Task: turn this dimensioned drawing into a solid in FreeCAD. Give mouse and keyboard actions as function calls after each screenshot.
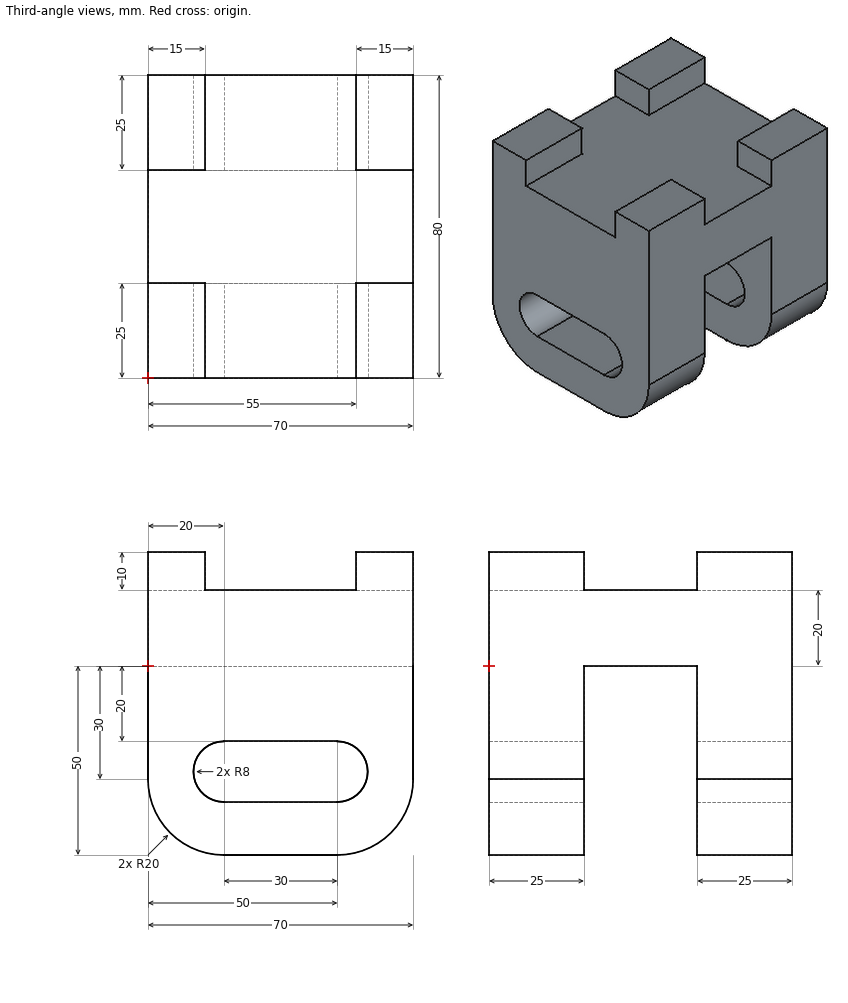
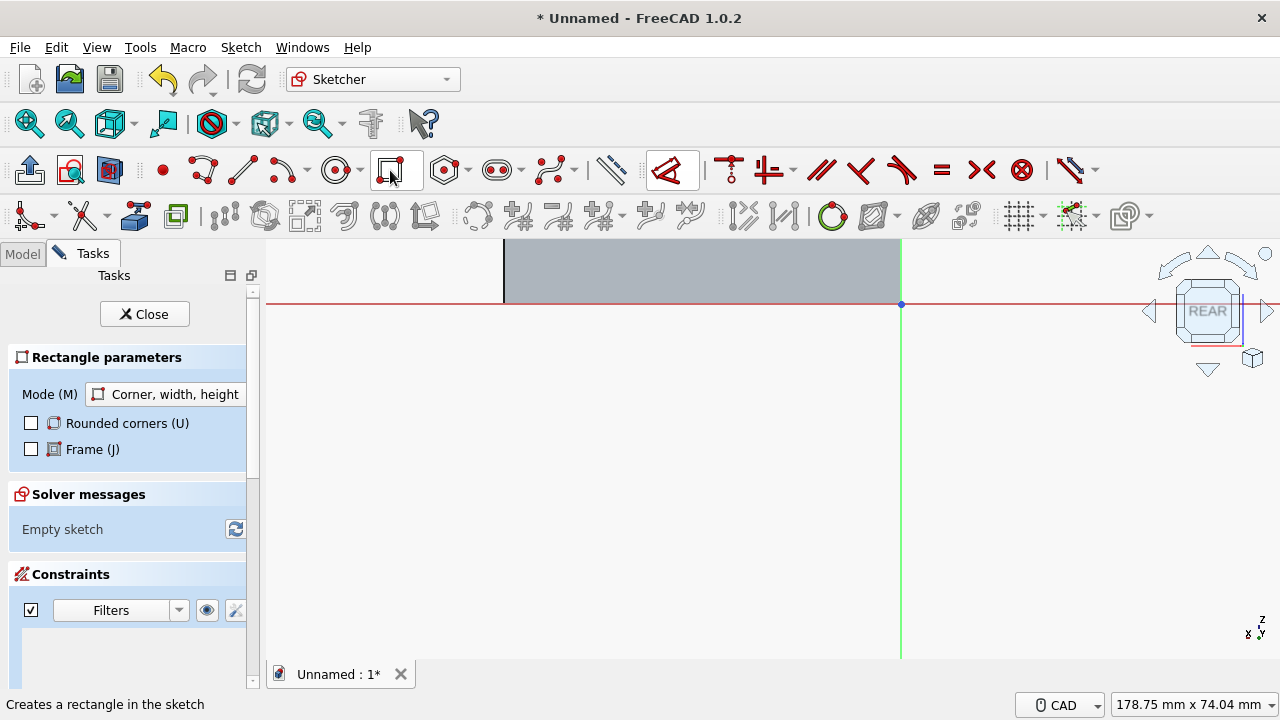
click(901, 304)
move(504, 588)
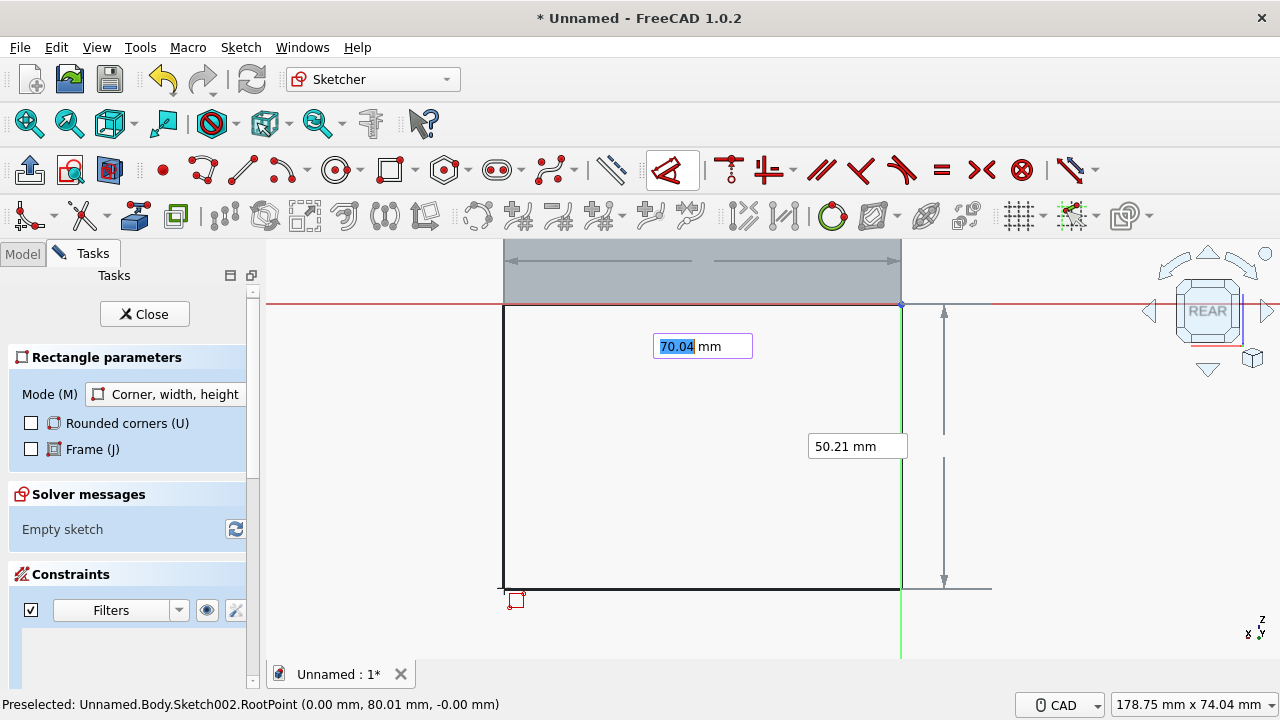
text(70)
key(Tab)
text(50)
key(Return)
key(Escape)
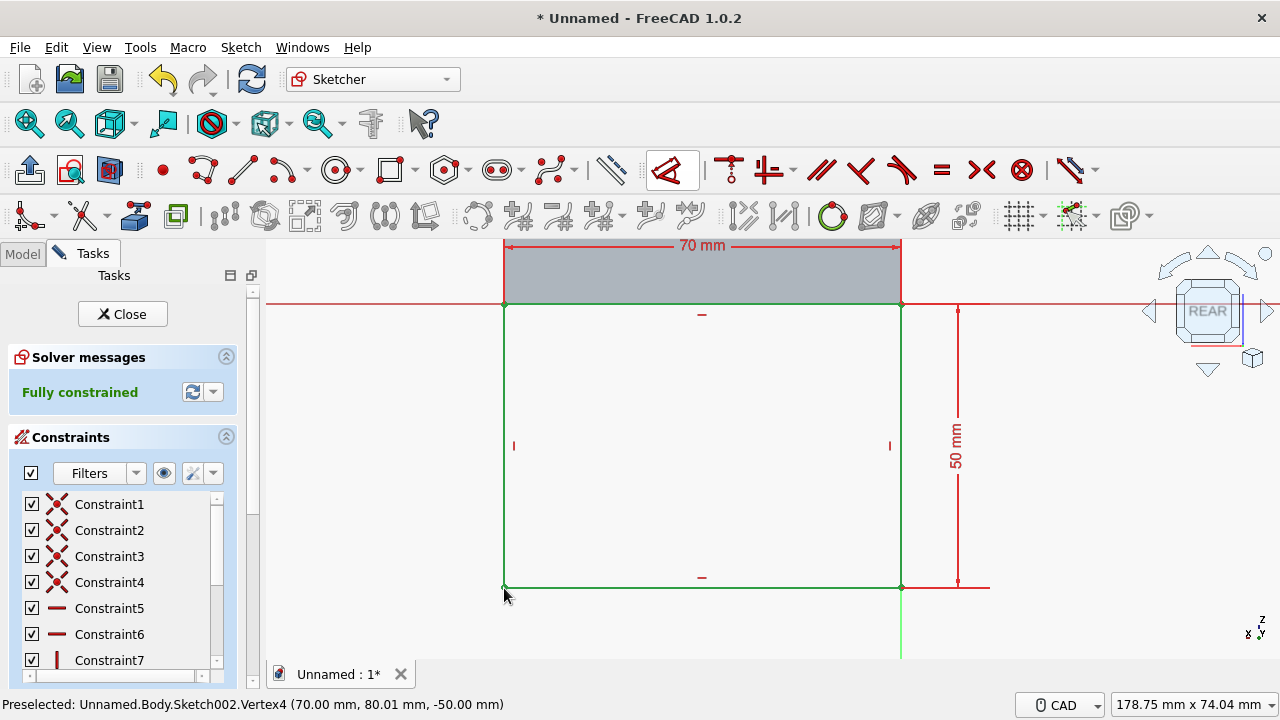
click(123, 314)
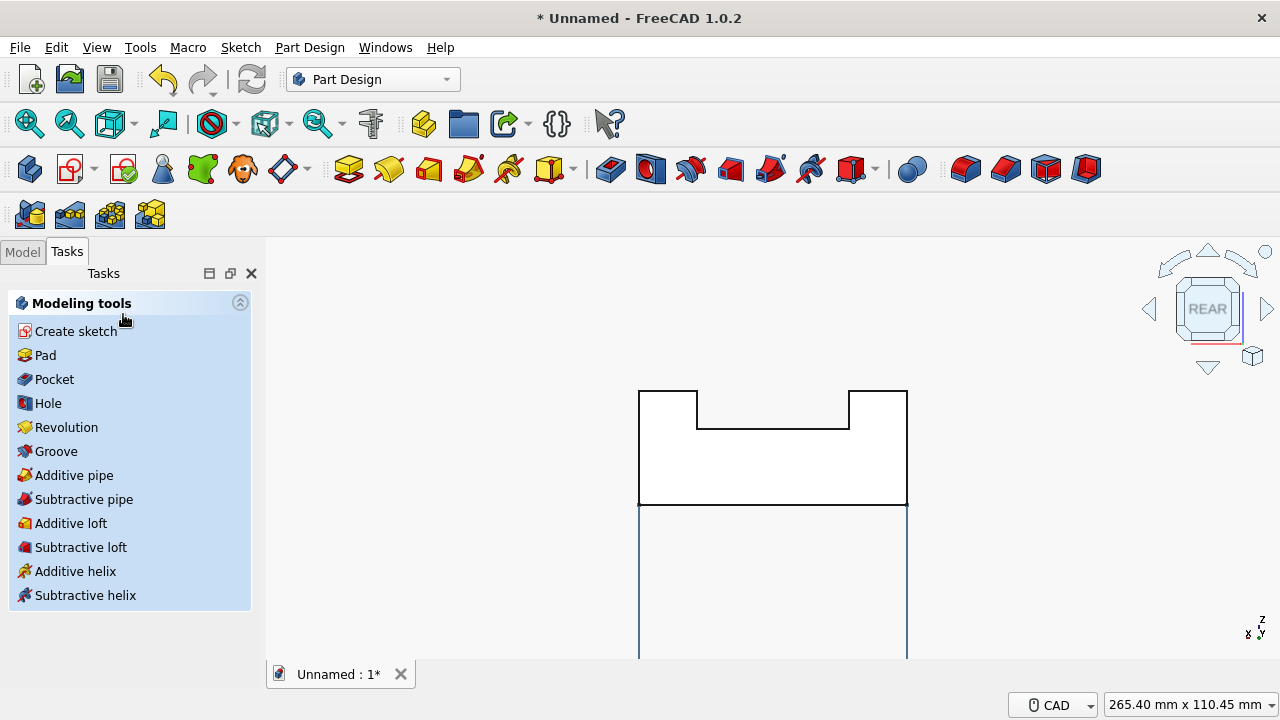
click(350, 170)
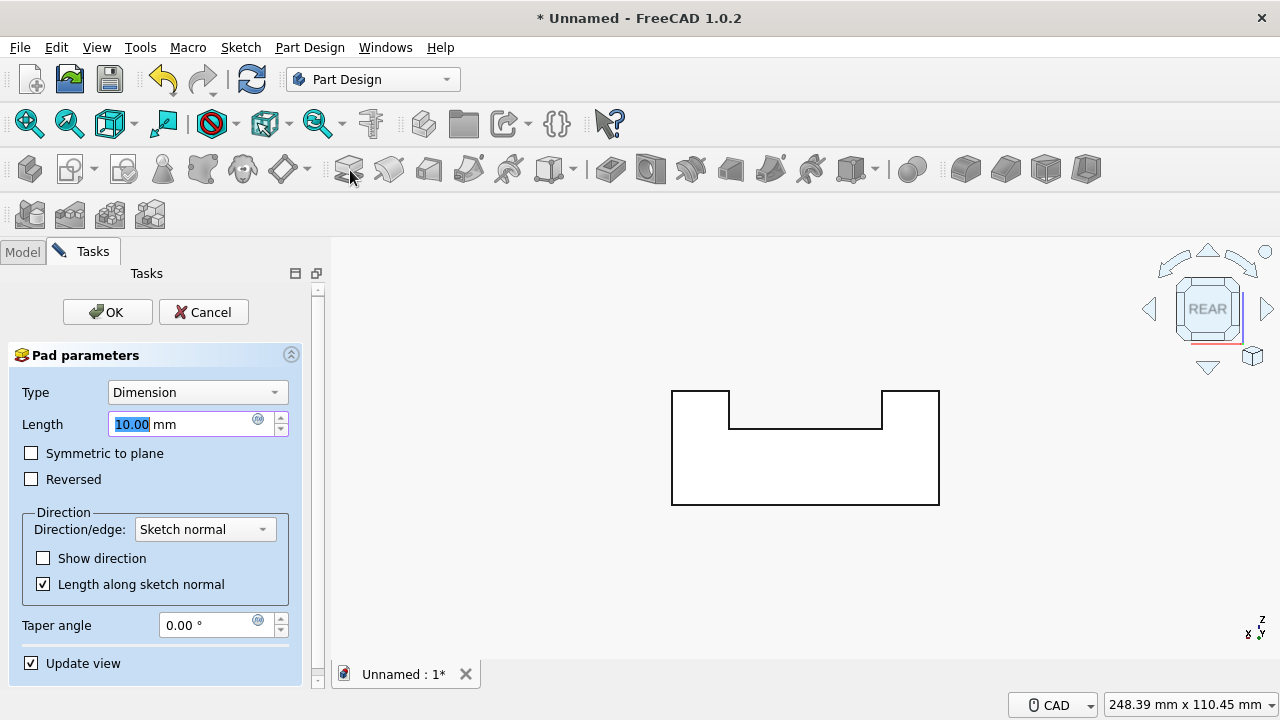
text(25)
key(Tab)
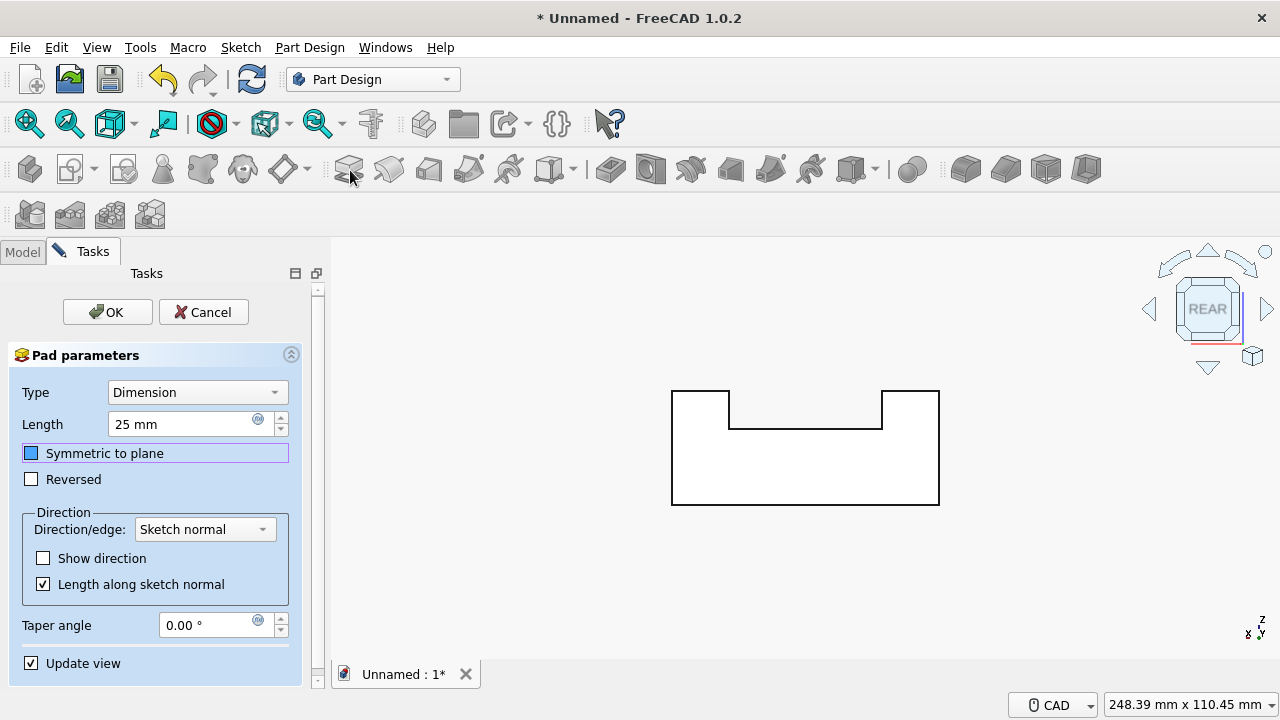
click(30, 479)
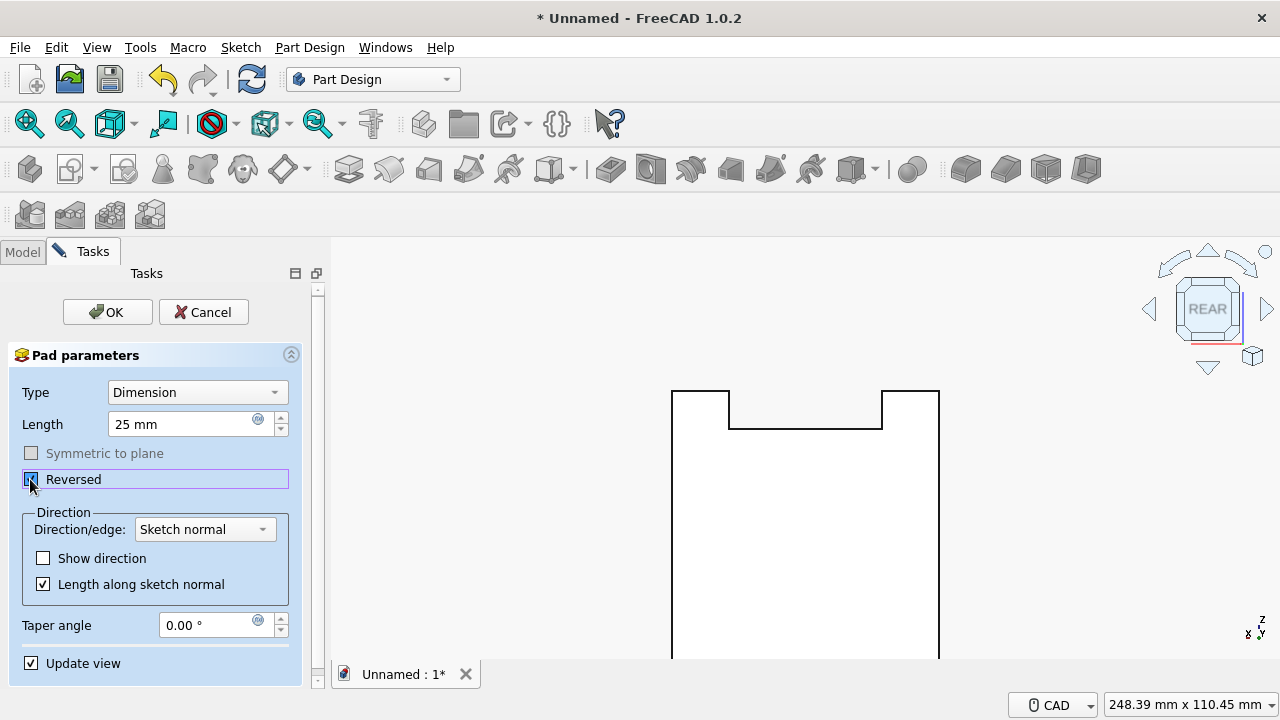
click(108, 312)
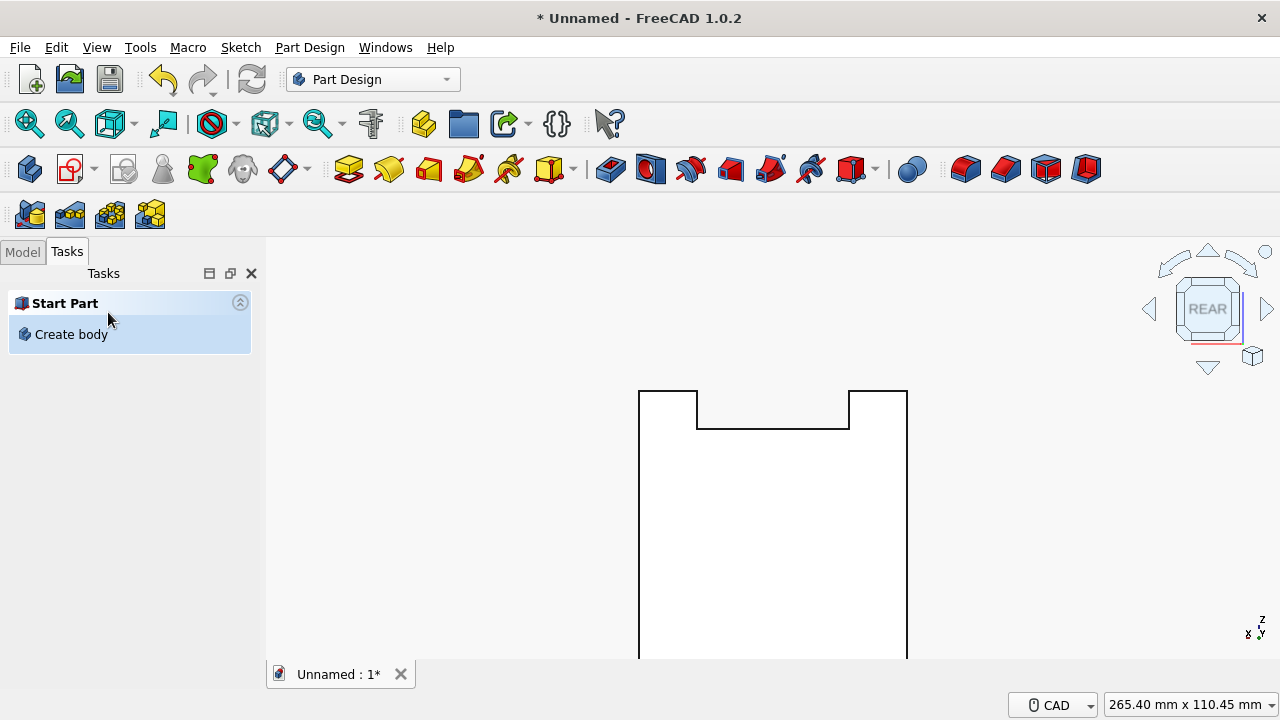
click(30, 124)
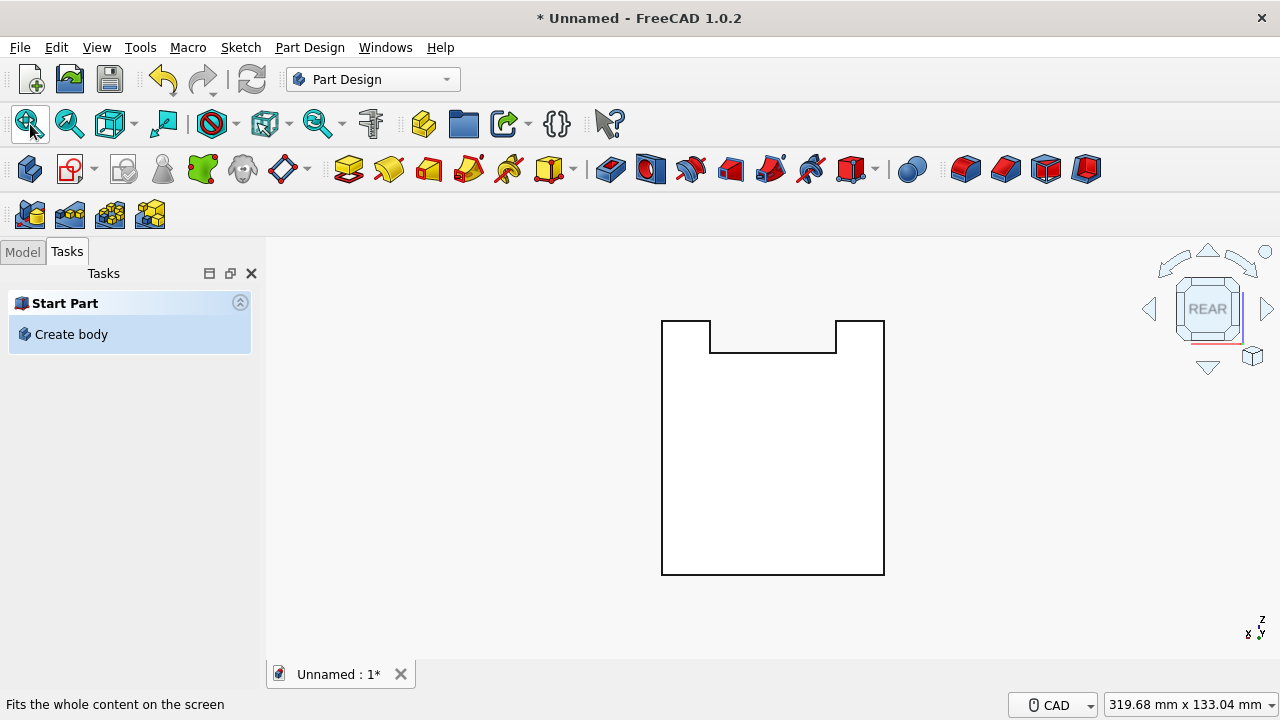
click(70, 170)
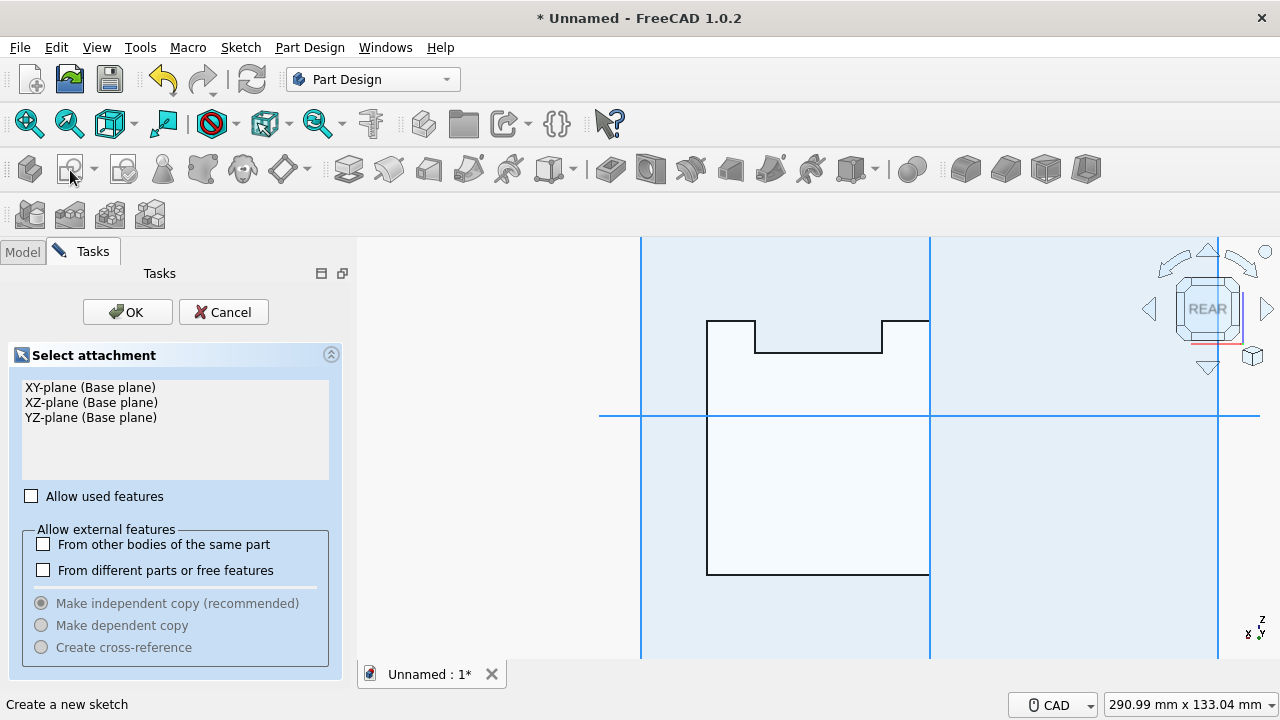
click(82, 402)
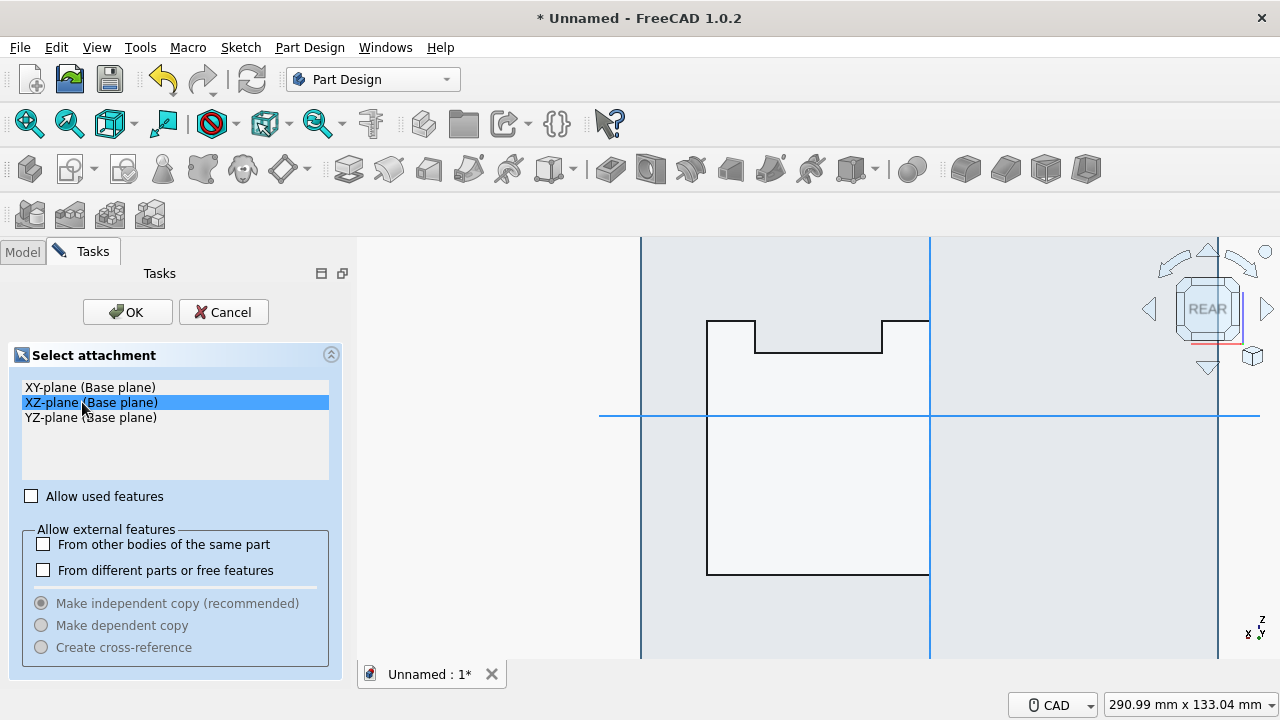
click(128, 312)